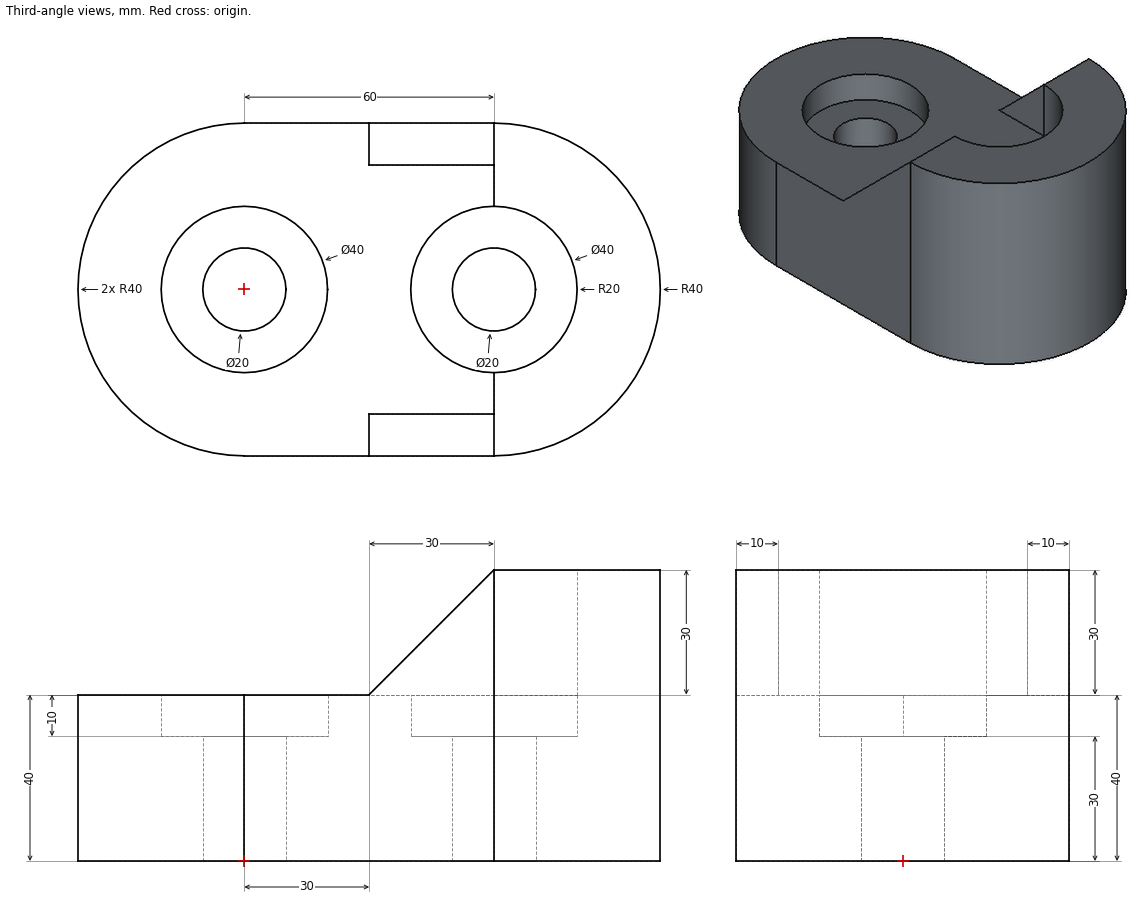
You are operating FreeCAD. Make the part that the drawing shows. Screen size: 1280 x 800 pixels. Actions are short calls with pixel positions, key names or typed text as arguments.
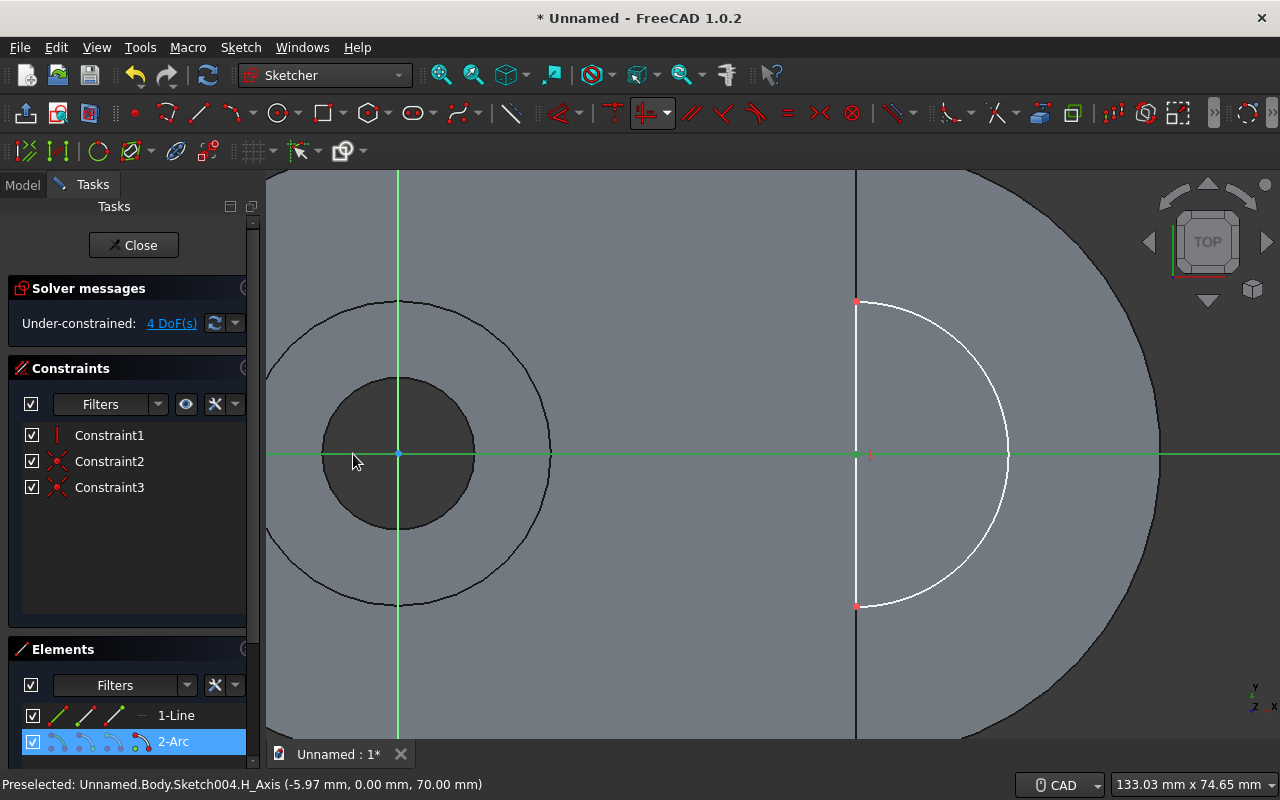
click(614, 114)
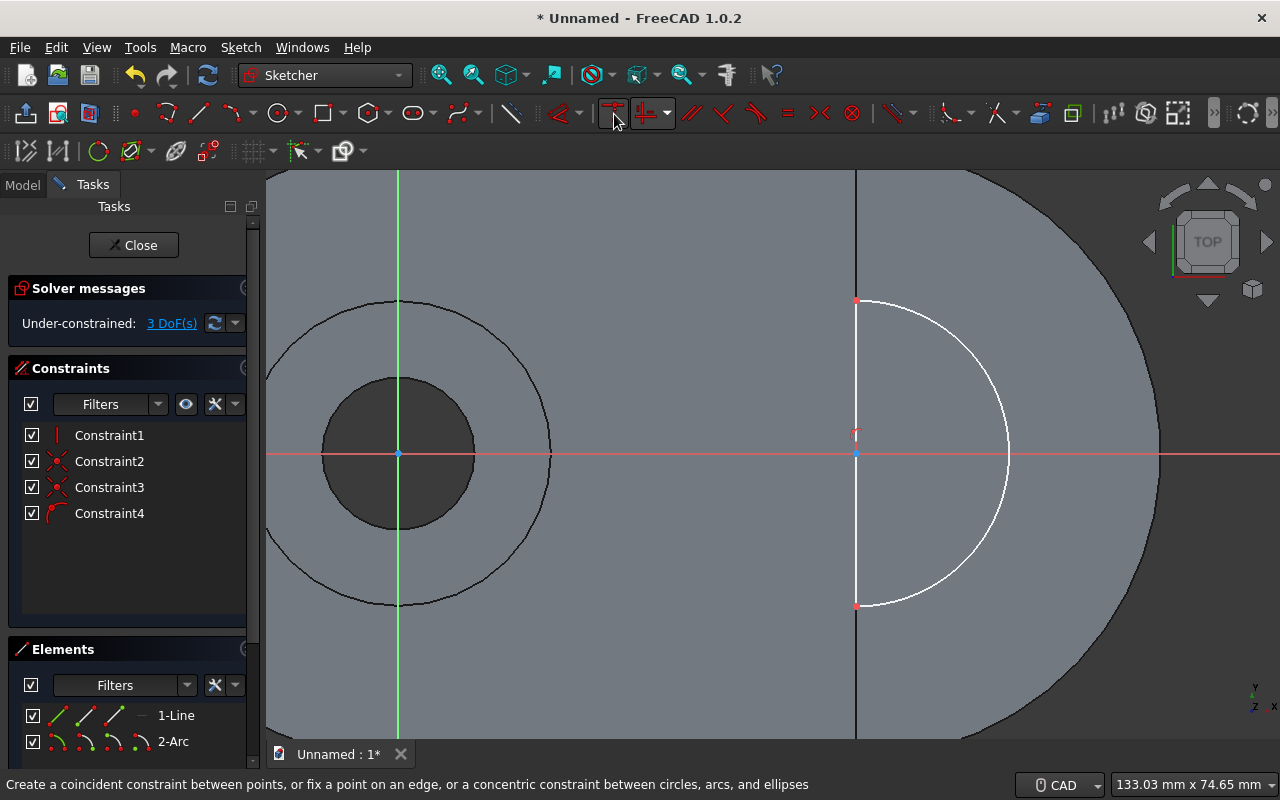
click(558, 114)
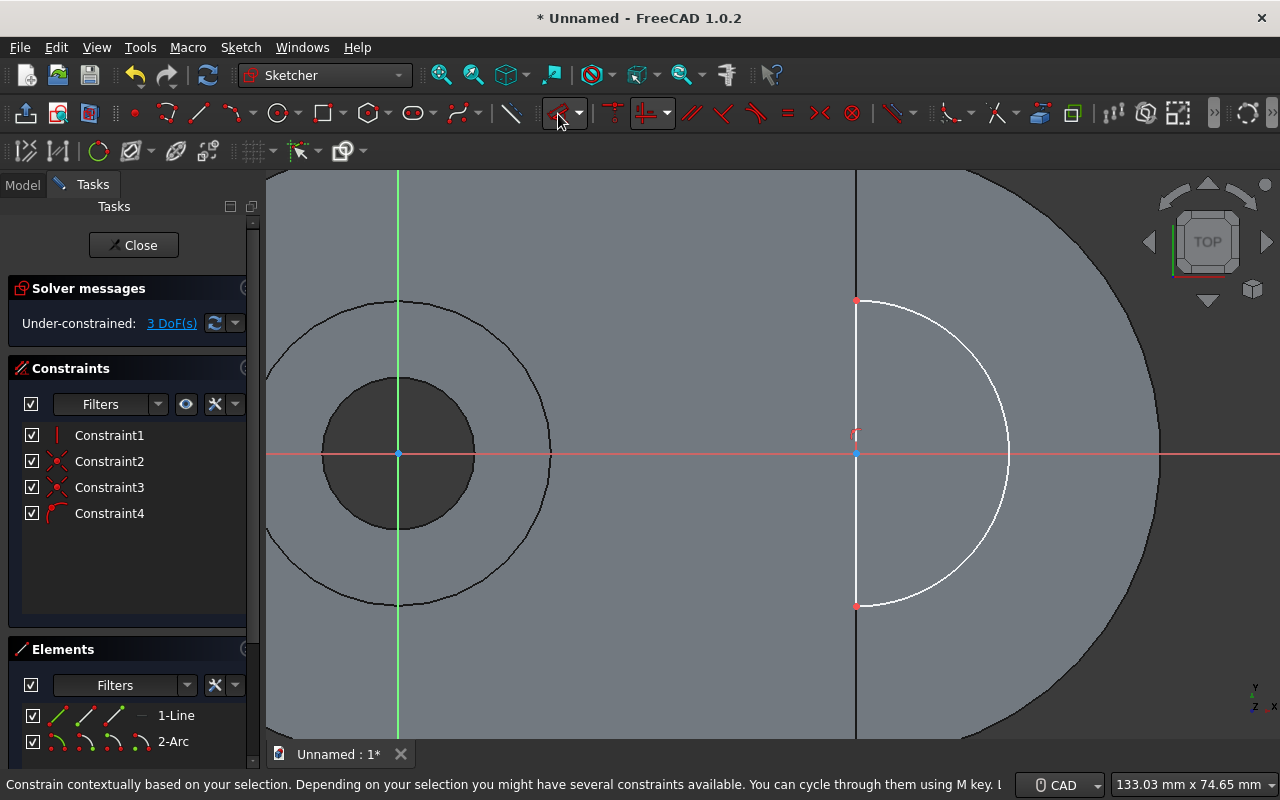
click(980, 543)
click(1006, 562)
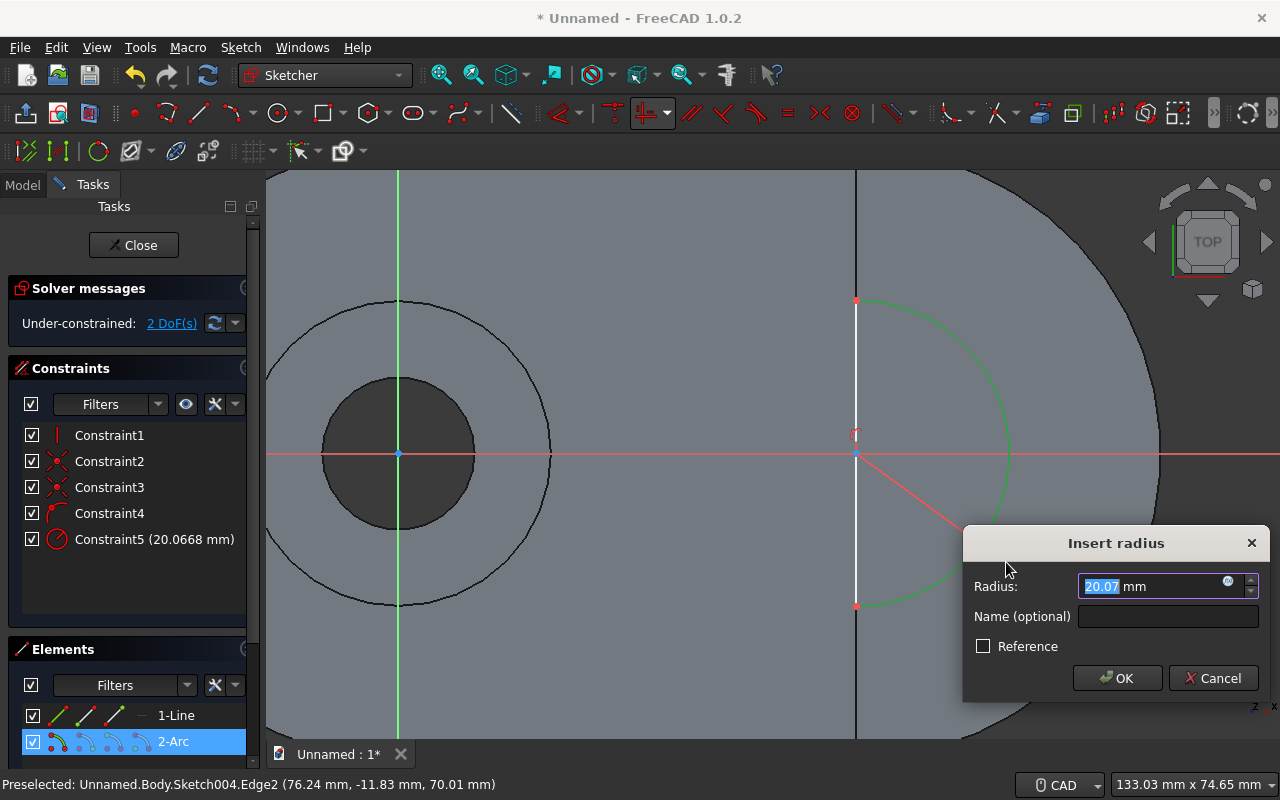
text(20)
key(Return)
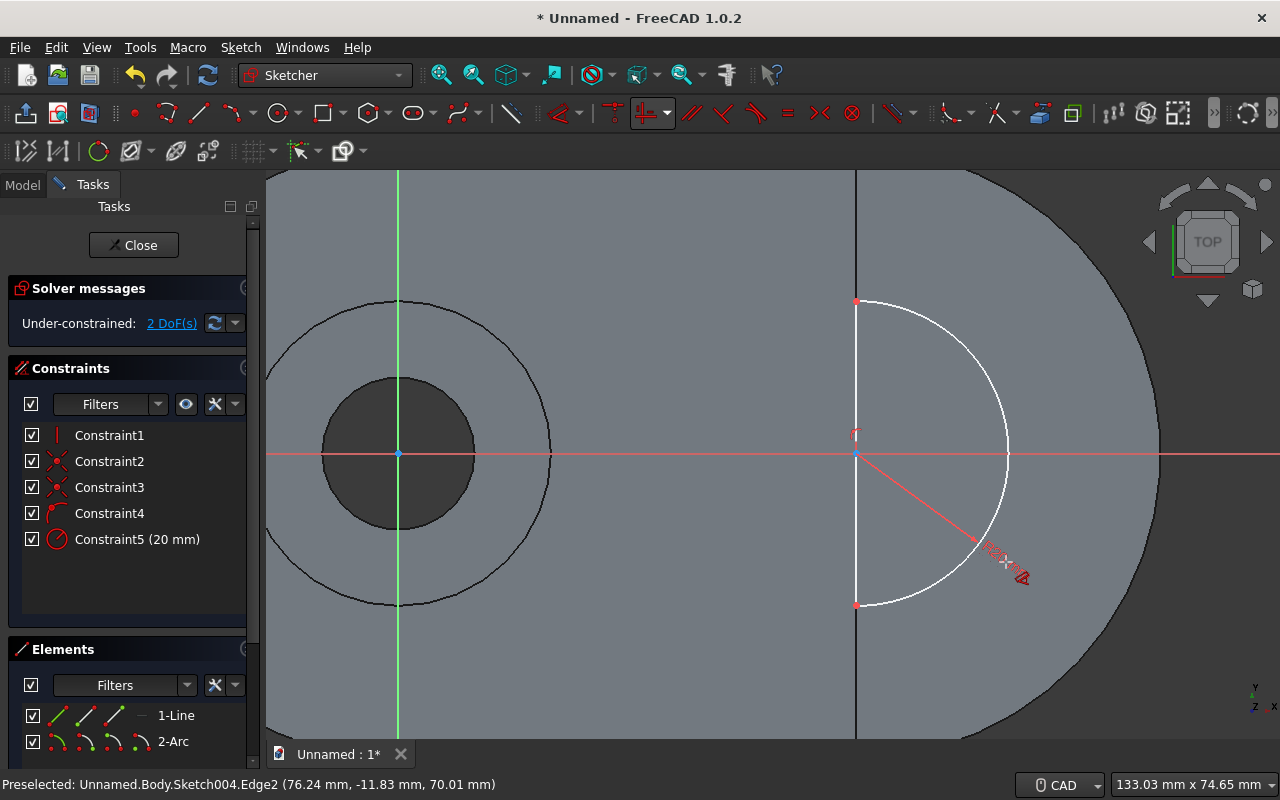
click(856, 301)
click(627, 267)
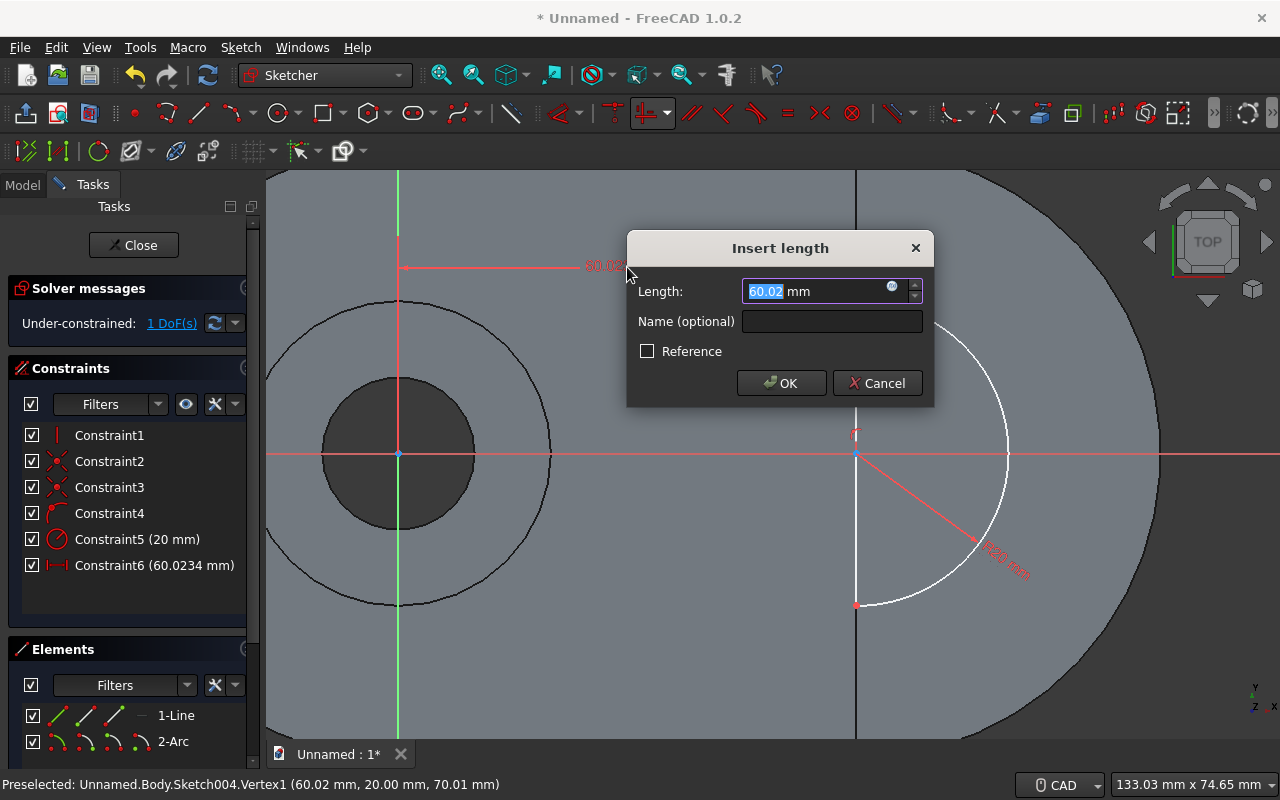
text(60)
key(Return)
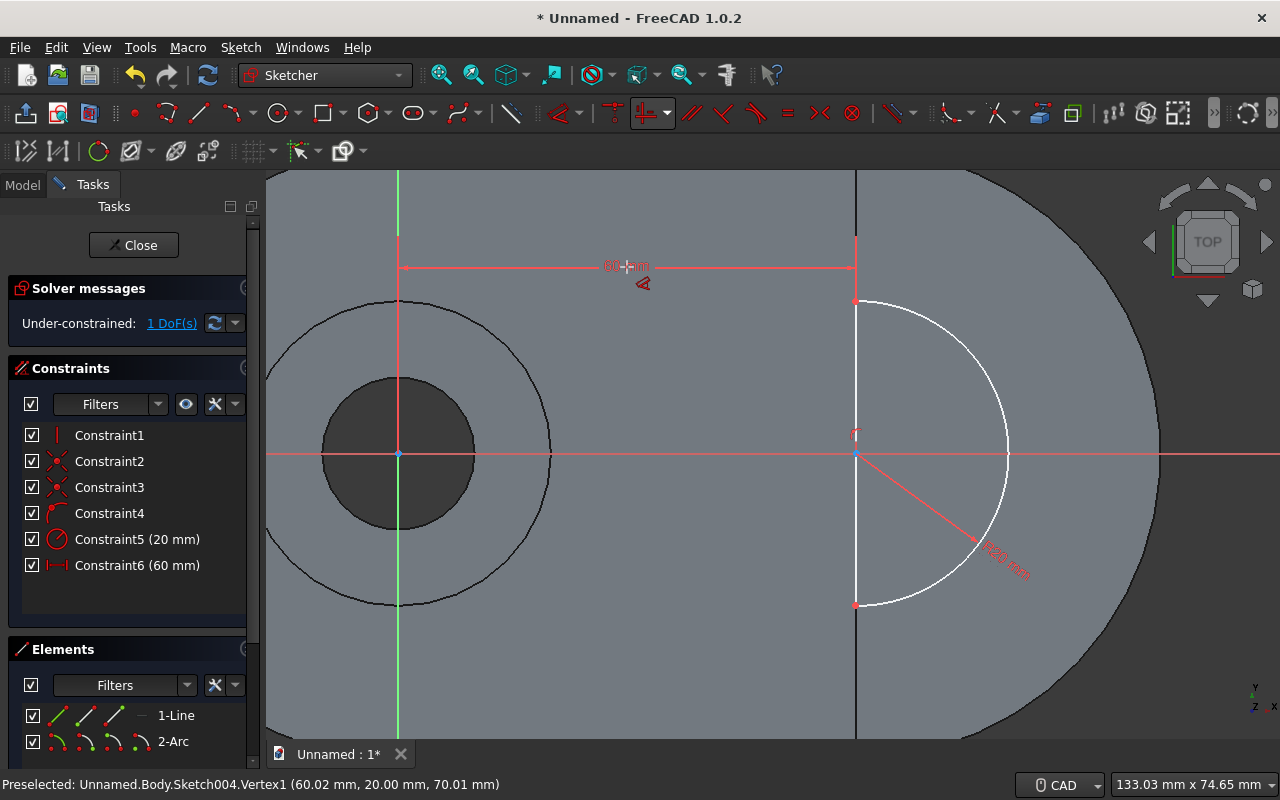
click(856, 454)
click(627, 488)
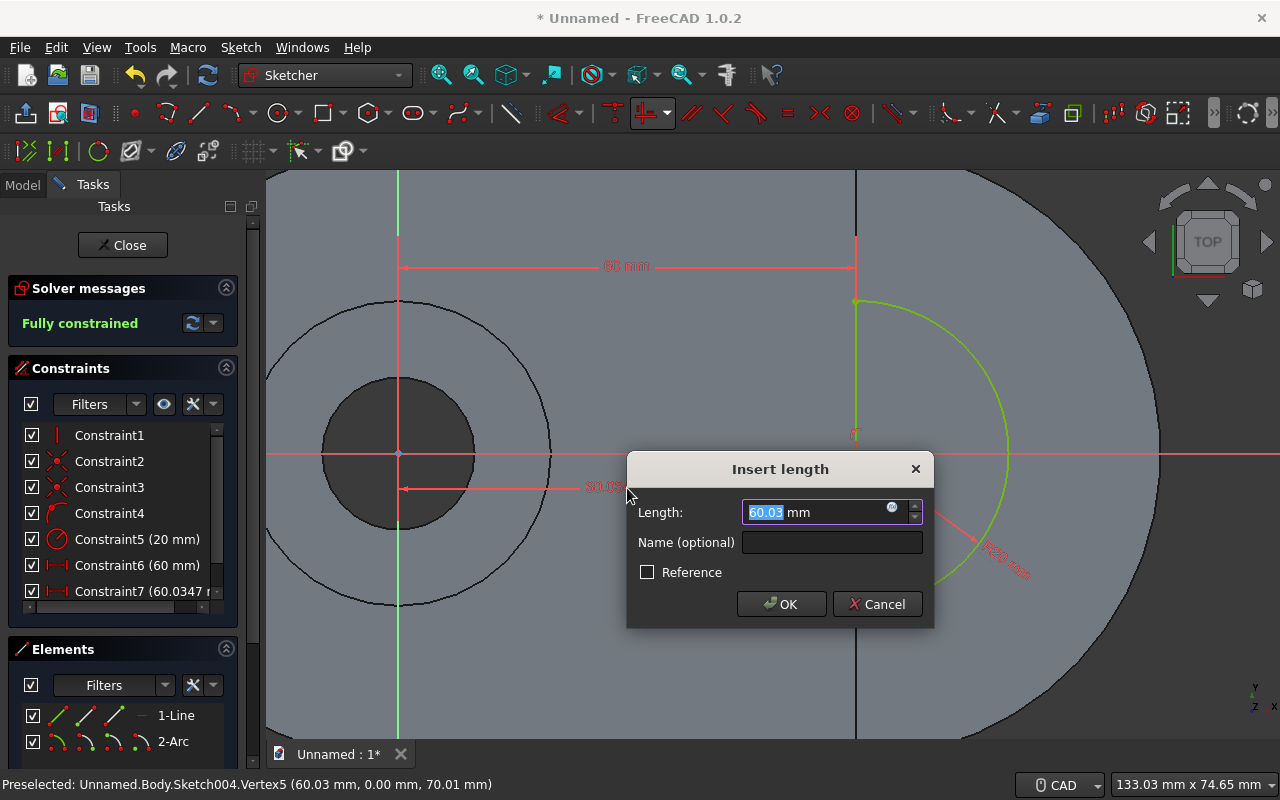
text(60)
key(Return)
key(Escape)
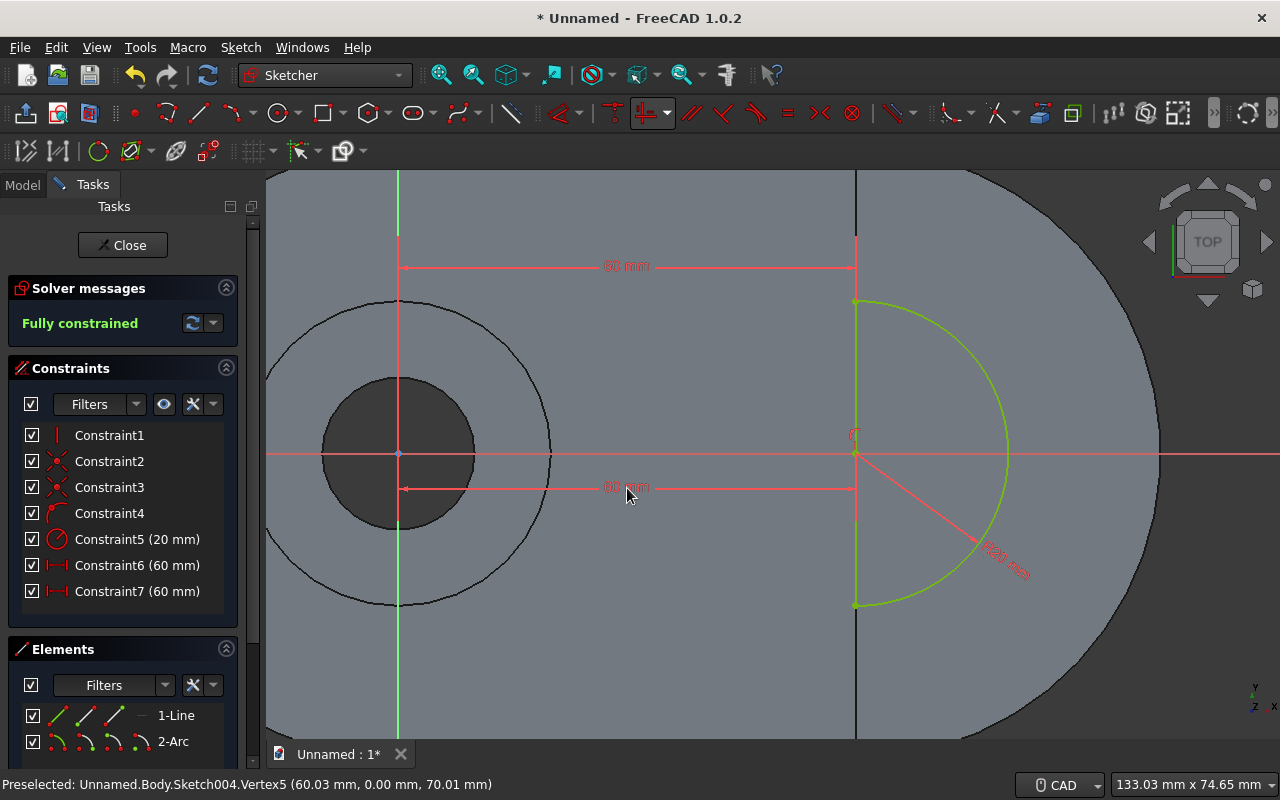
click(123, 245)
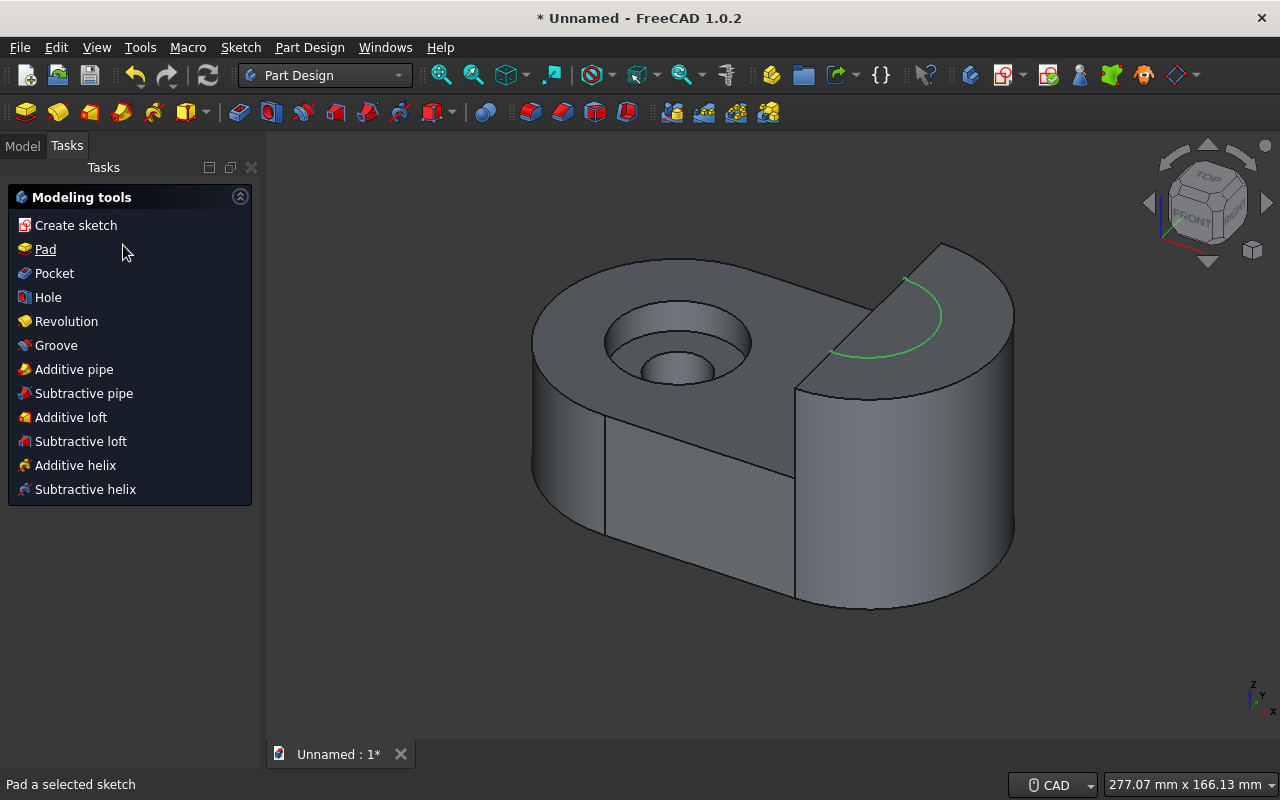
click(240, 112)